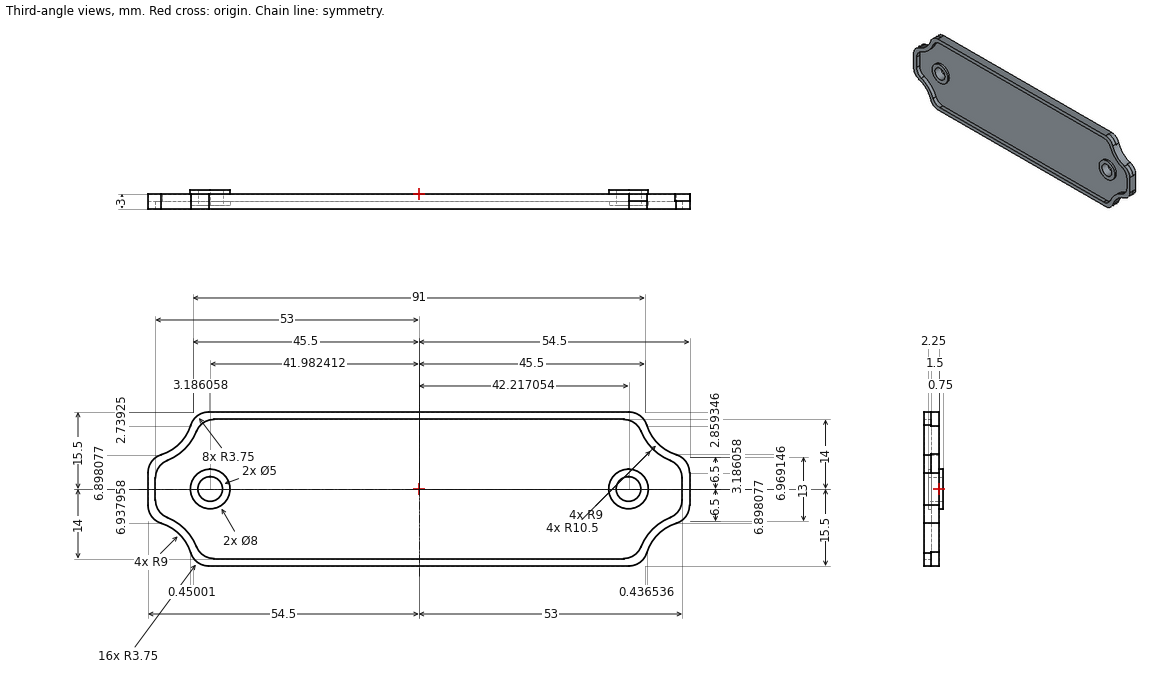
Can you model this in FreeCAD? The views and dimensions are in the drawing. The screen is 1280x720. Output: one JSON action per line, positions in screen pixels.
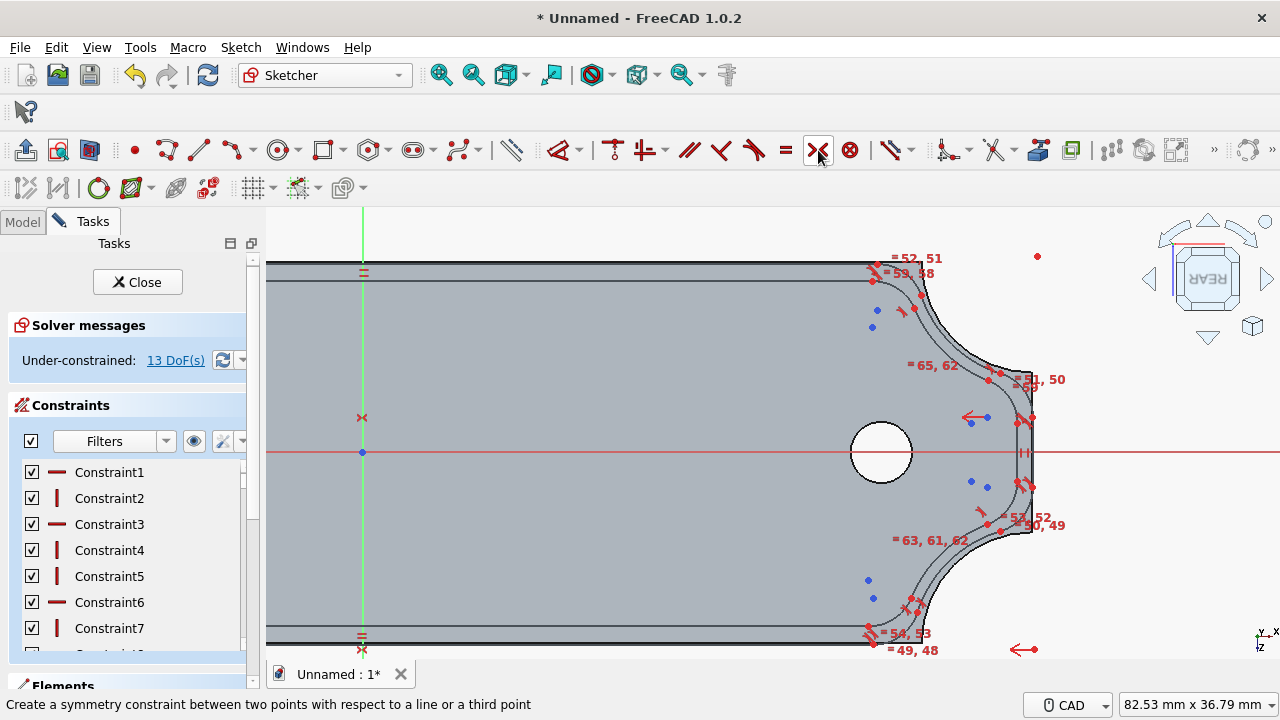
{"action": "left_click", "coordinate": [874, 599]}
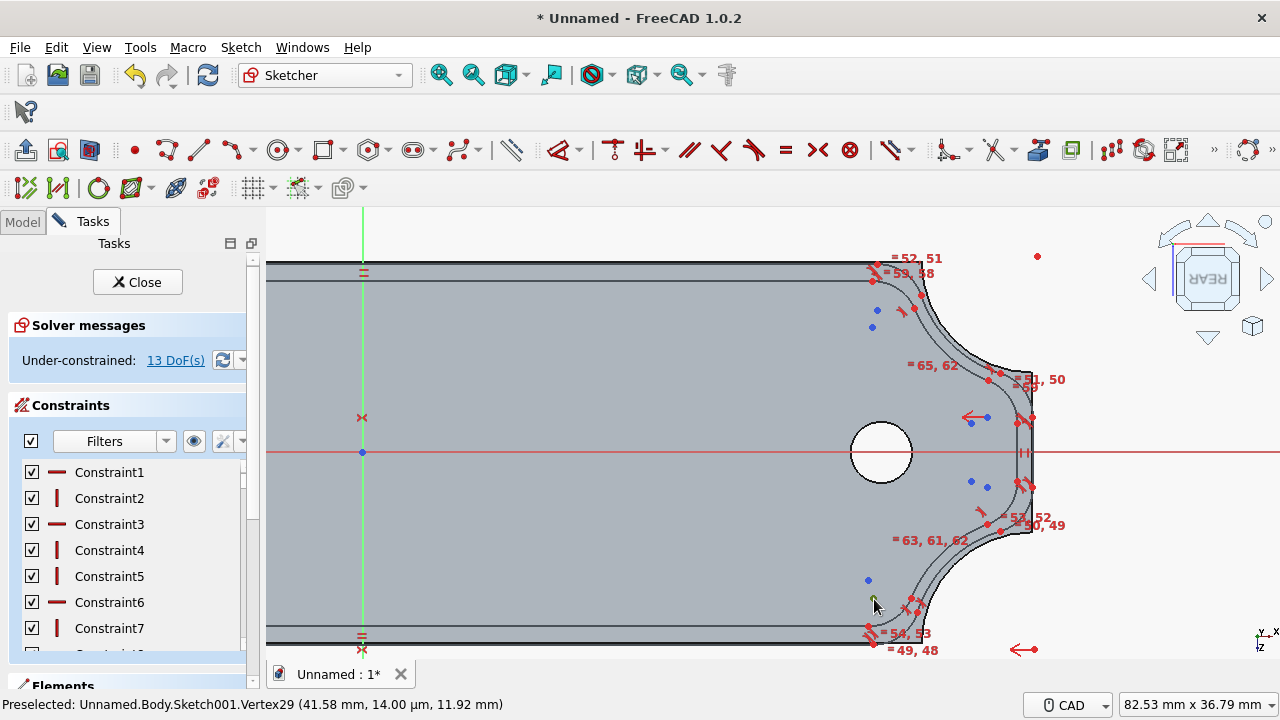
{"action": "left_click", "coordinate": [878, 310]}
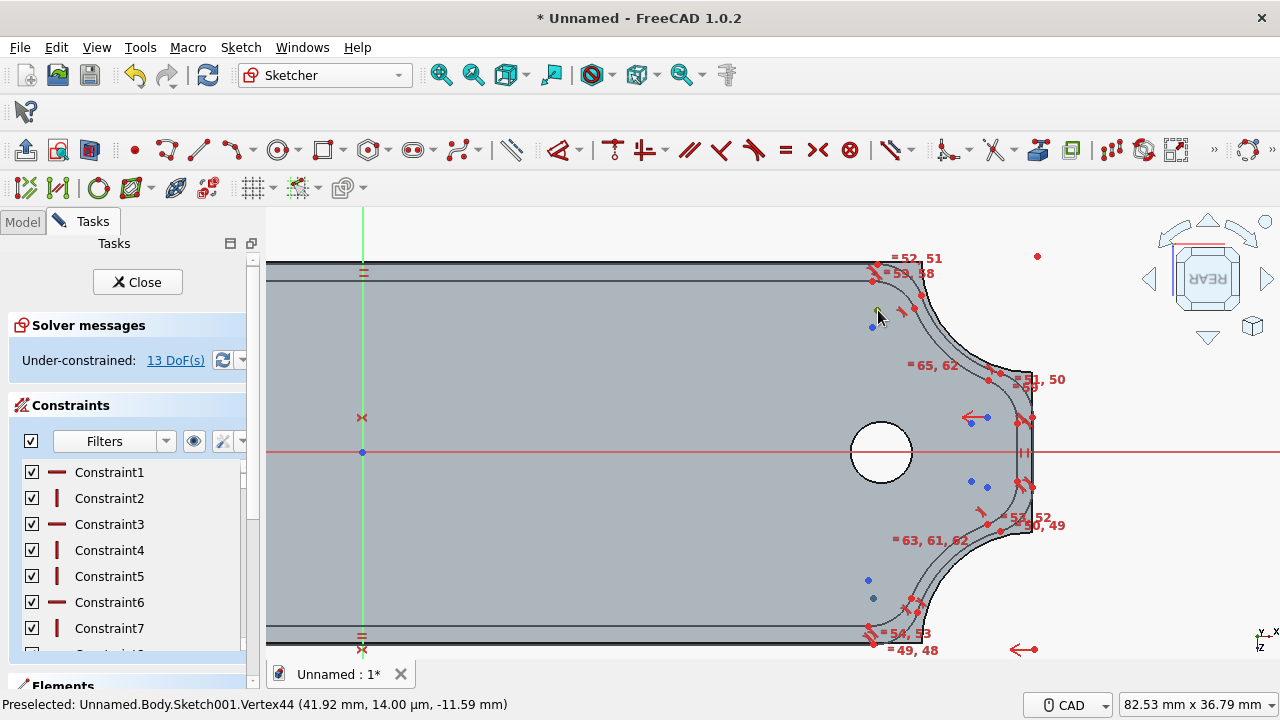
{"action": "left_click", "coordinate": [411, 452]}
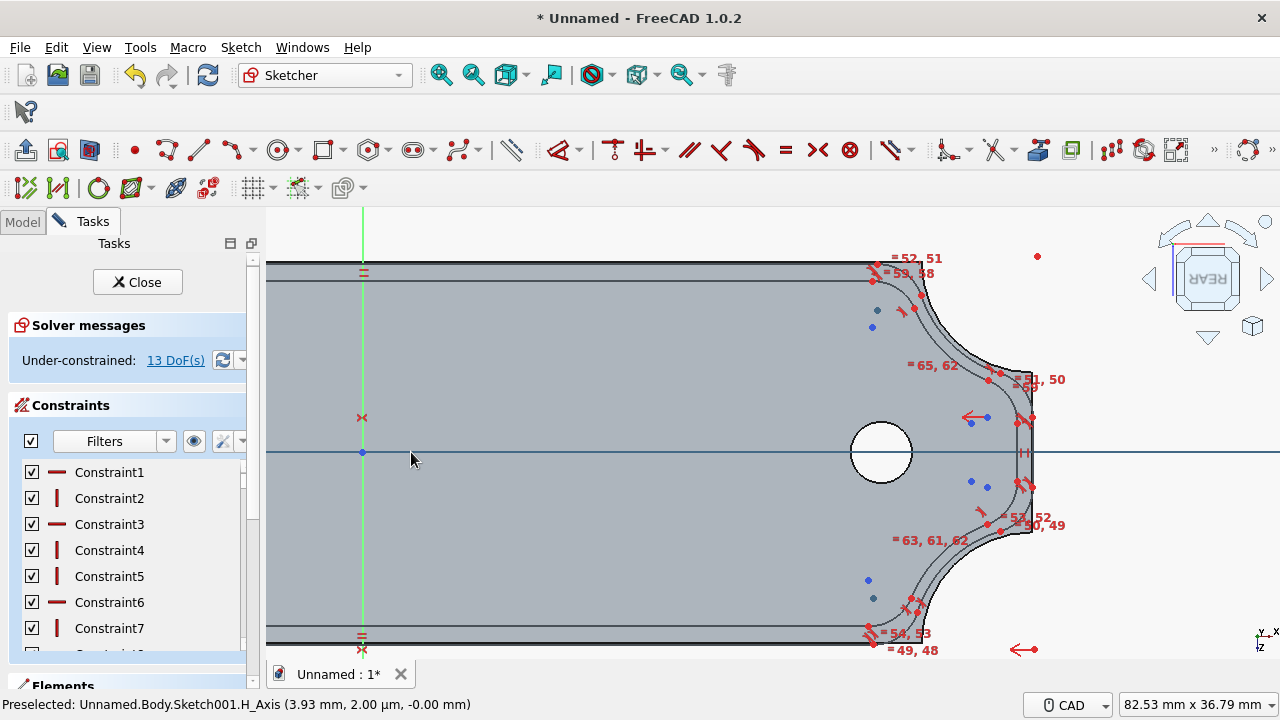
{"action": "left_click", "coordinate": [818, 150]}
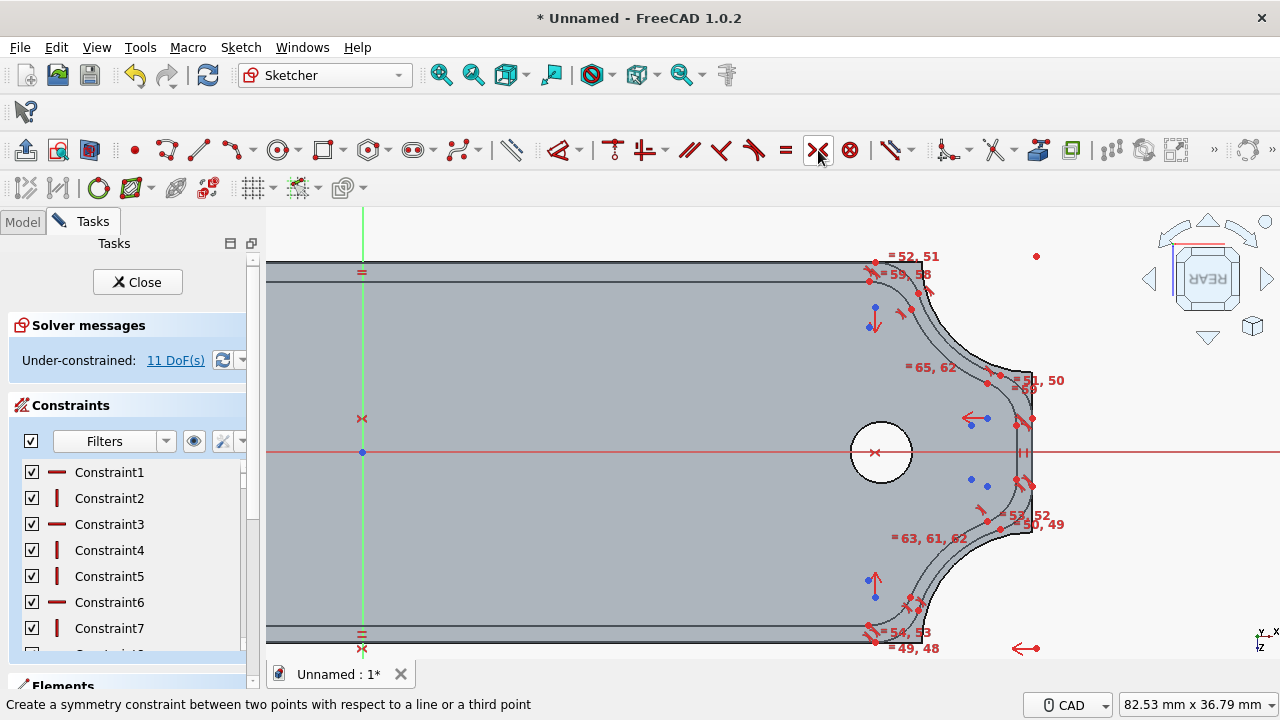
{"action": "left_click", "coordinate": [558, 150]}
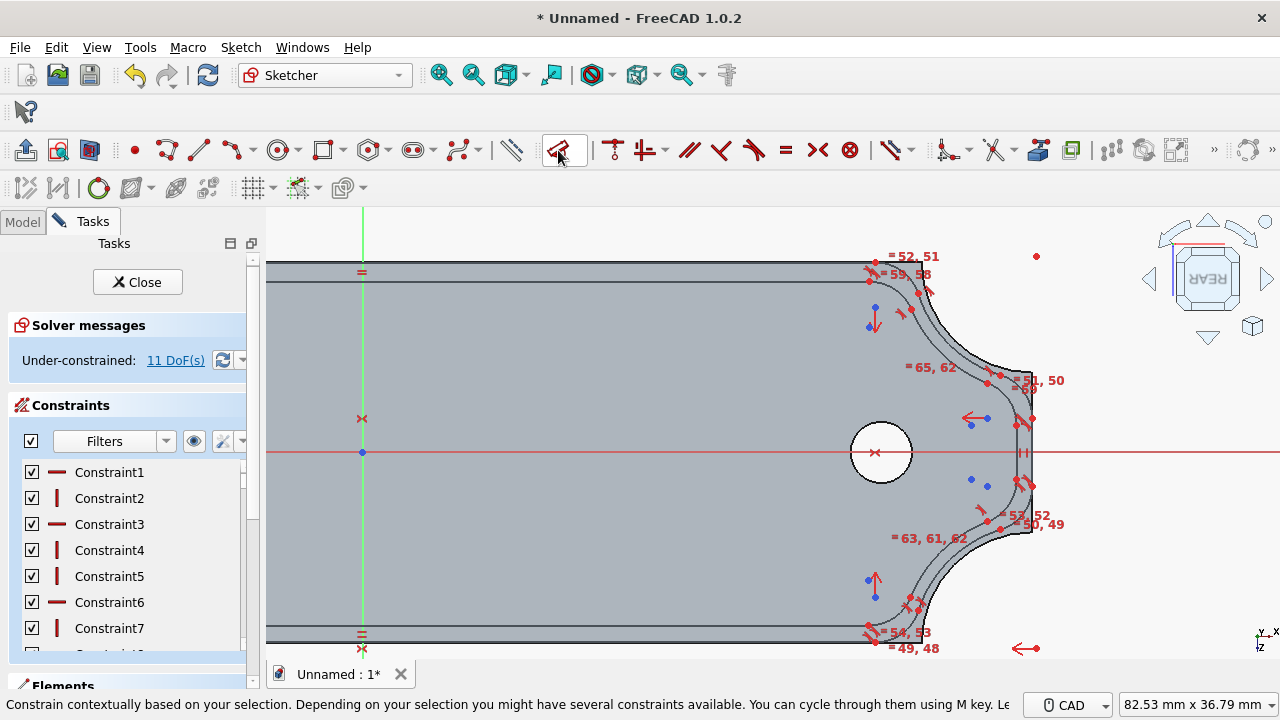
{"action": "scroll", "coordinate": [983, 417], "scroll_direction": "down", "scroll_amount": 4}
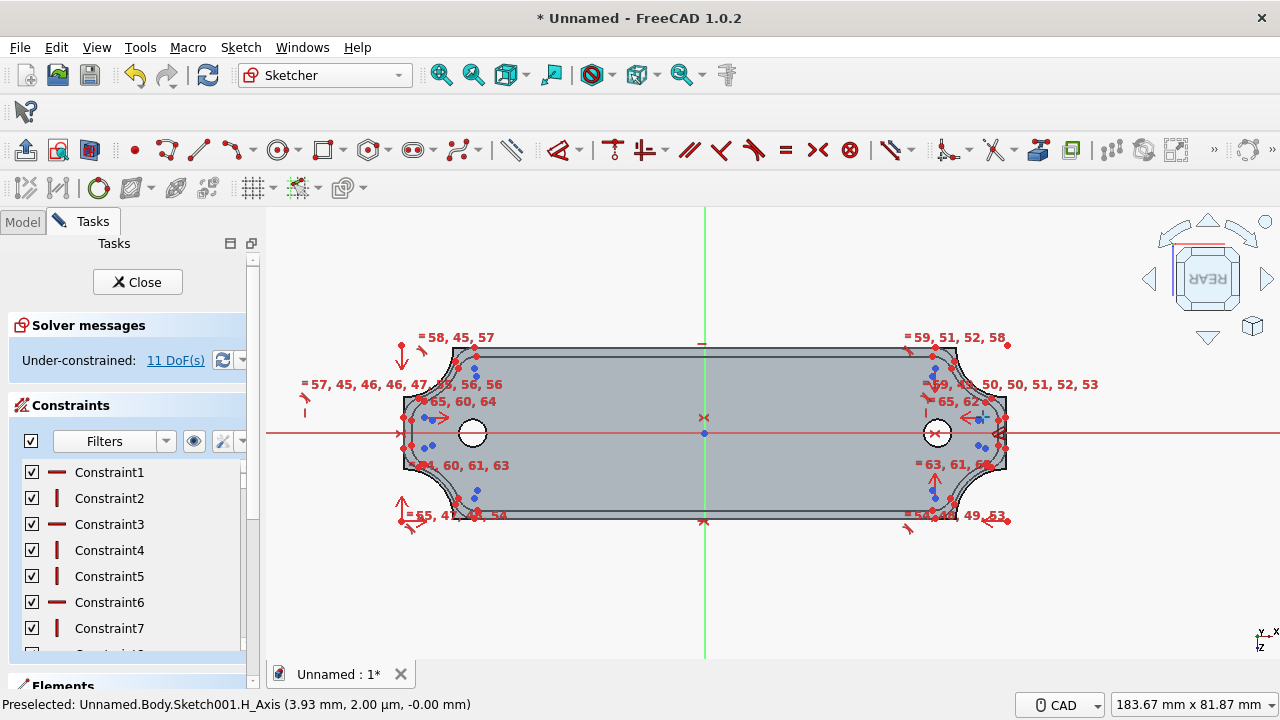
{"action": "scroll", "coordinate": [467, 349], "scroll_direction": "up", "scroll_amount": 4}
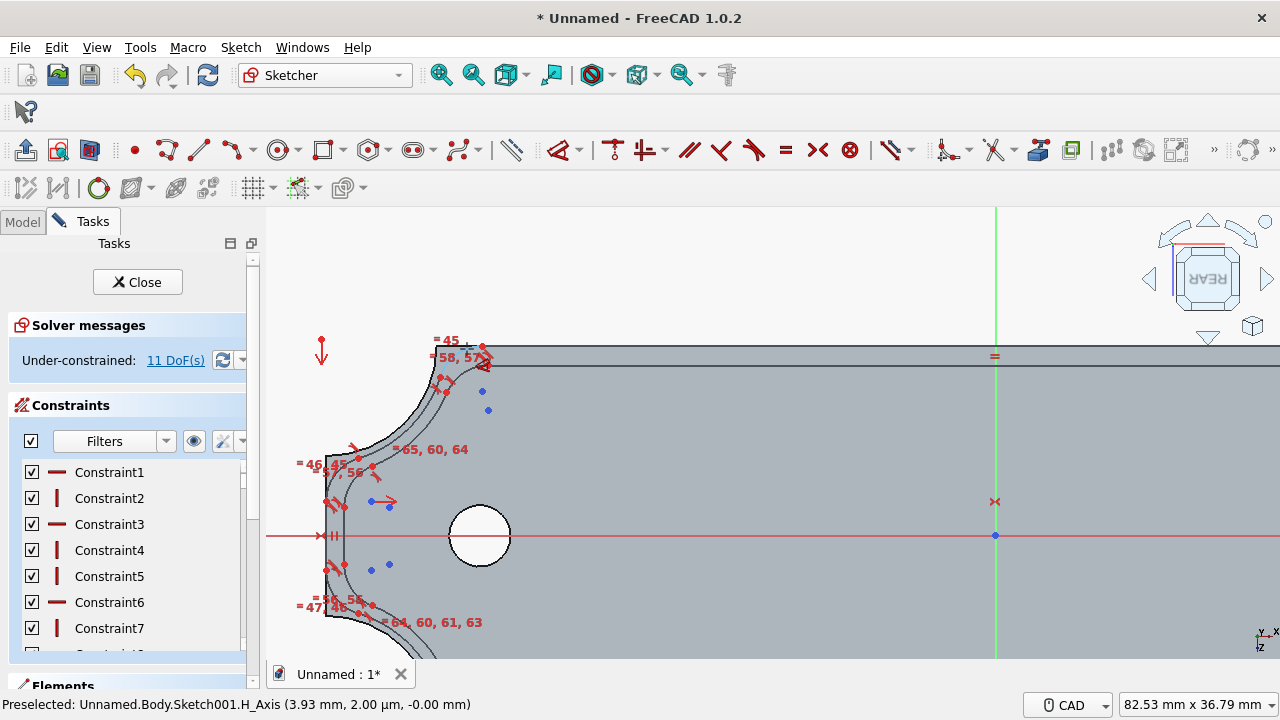
{"action": "left_click", "coordinate": [466, 349]}
{"action": "left_click", "coordinate": [454, 319]}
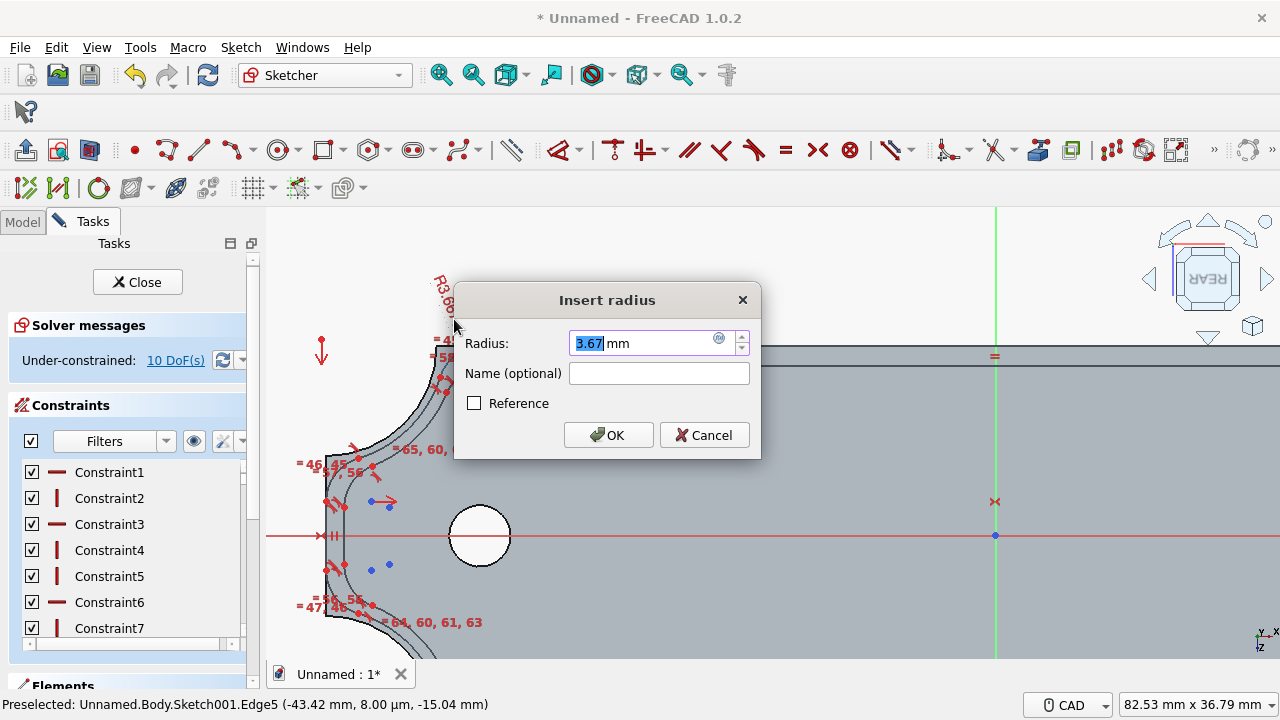
{"action": "type", "text": "3.75"}
{"action": "key", "text": "Return"}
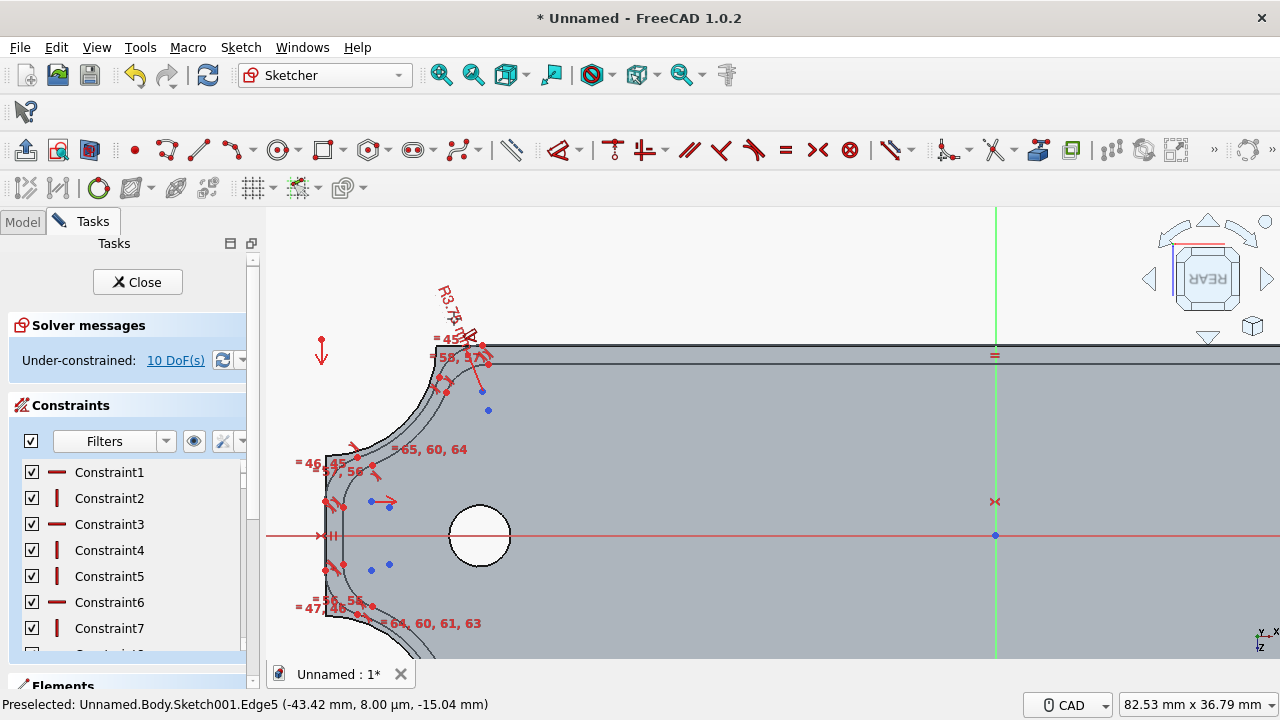
{"action": "left_click", "coordinate": [390, 442]}
{"action": "left_click", "coordinate": [408, 469]}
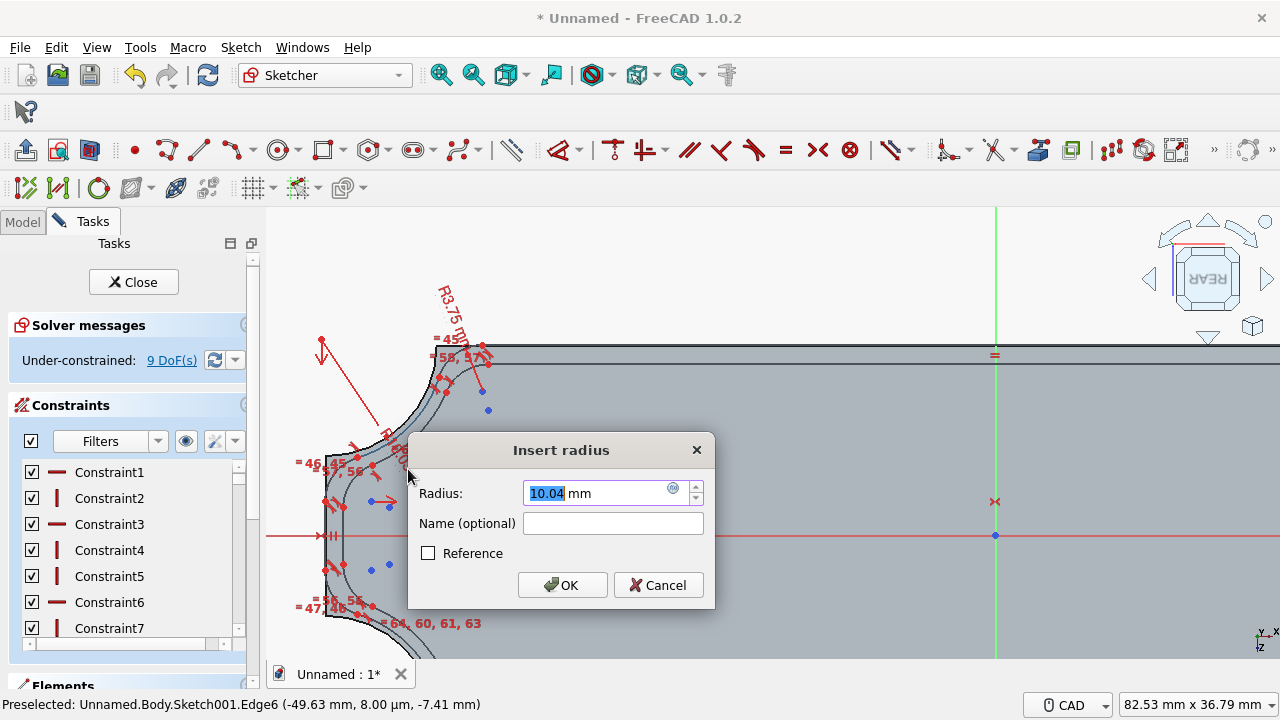
{"action": "type", "text": "9"}
{"action": "key", "text": "Return"}